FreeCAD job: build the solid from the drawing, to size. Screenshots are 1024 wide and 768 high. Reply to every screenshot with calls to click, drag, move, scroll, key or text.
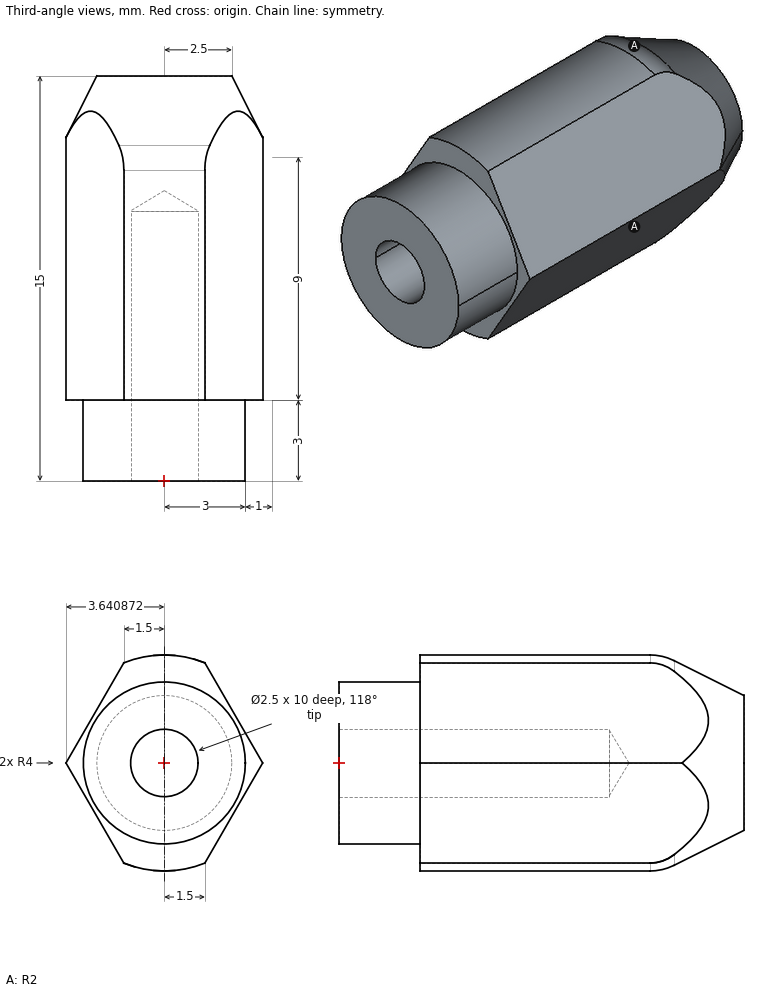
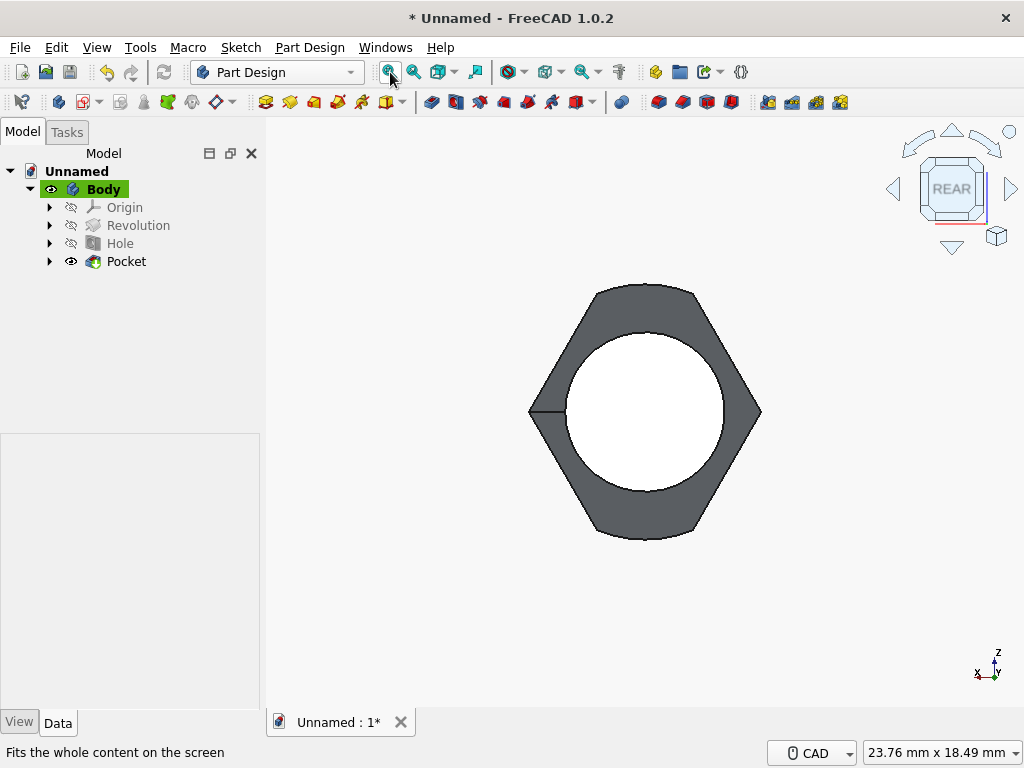
key(0)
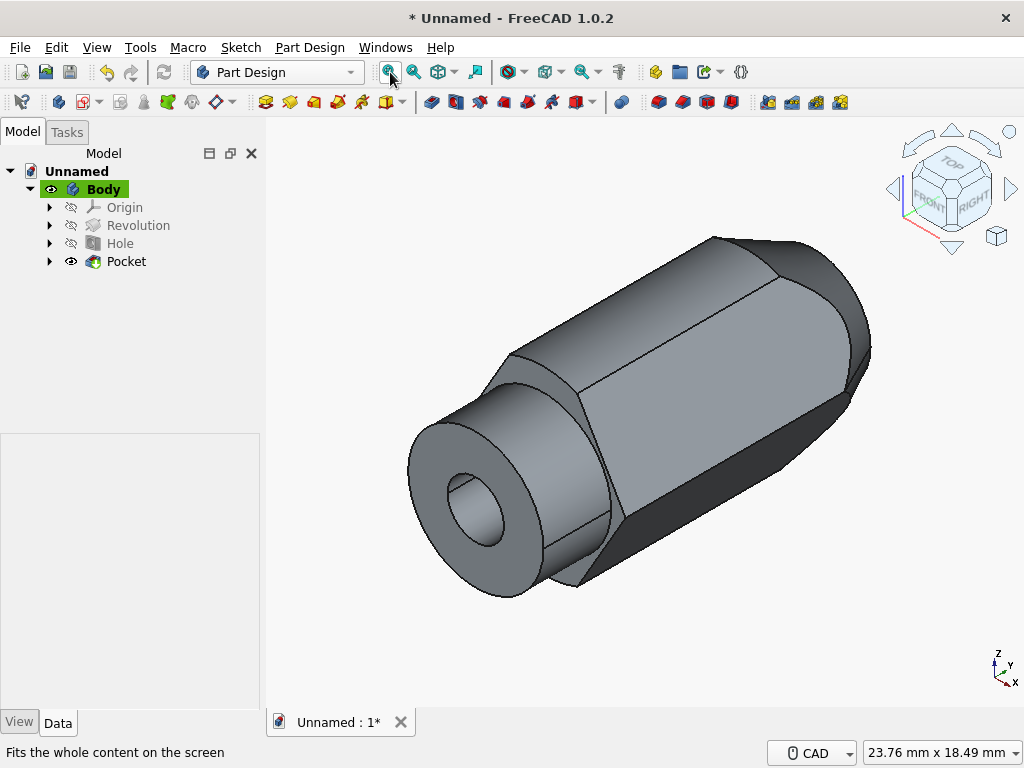
click(733, 241)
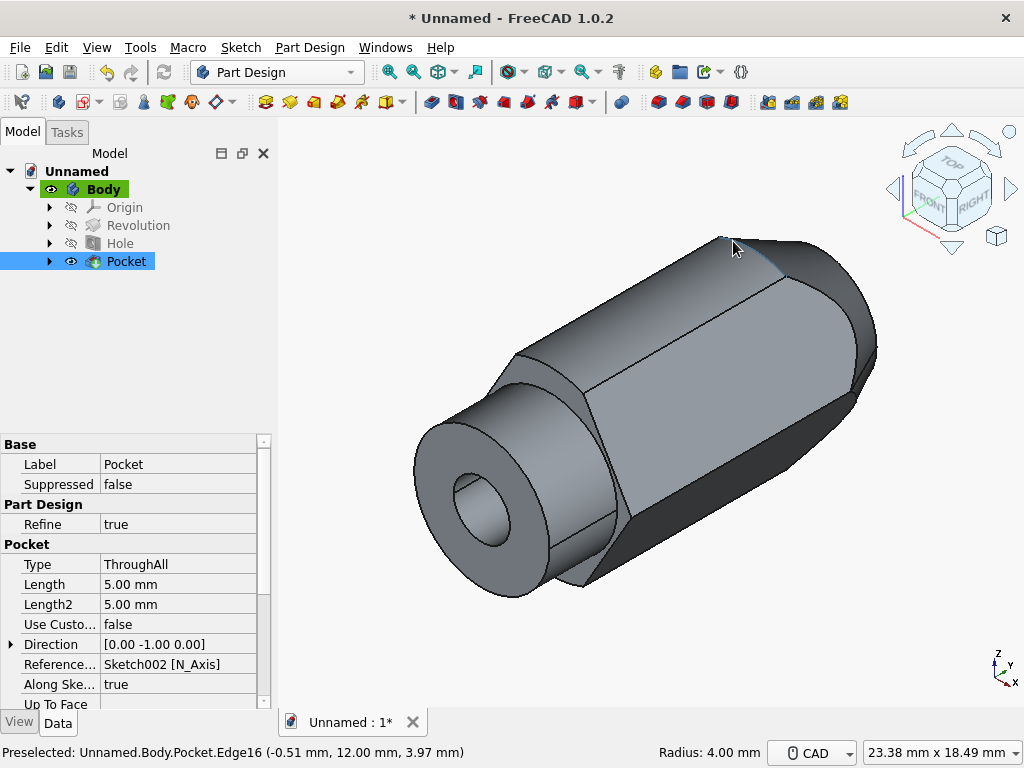
key(2)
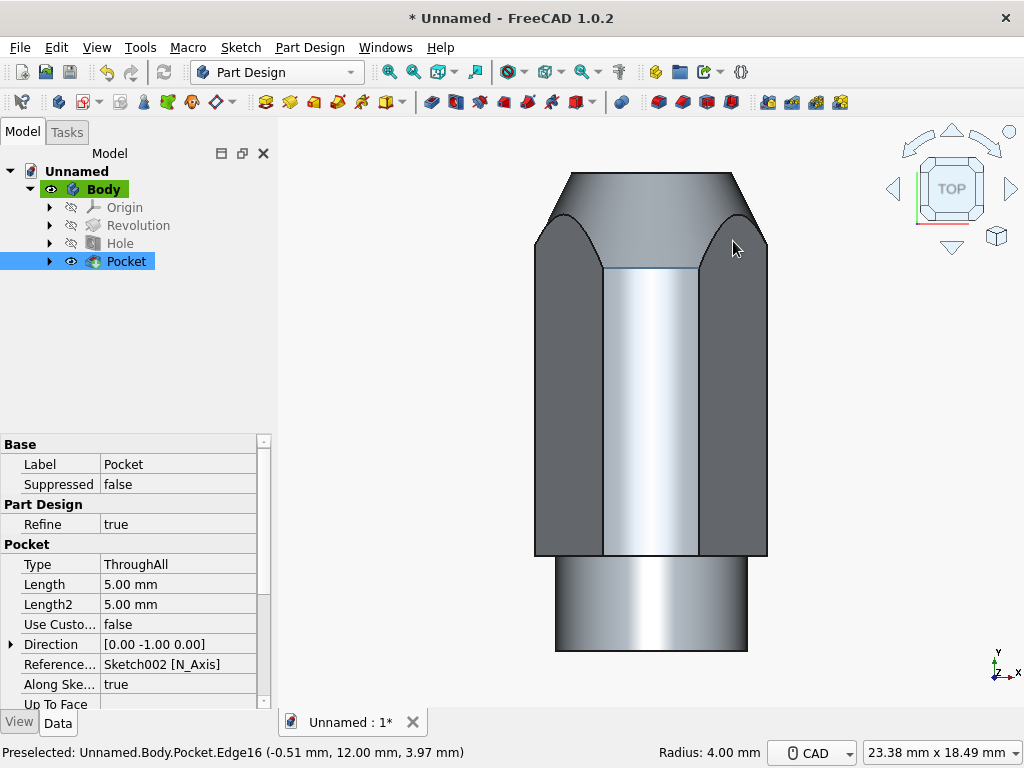
key(1)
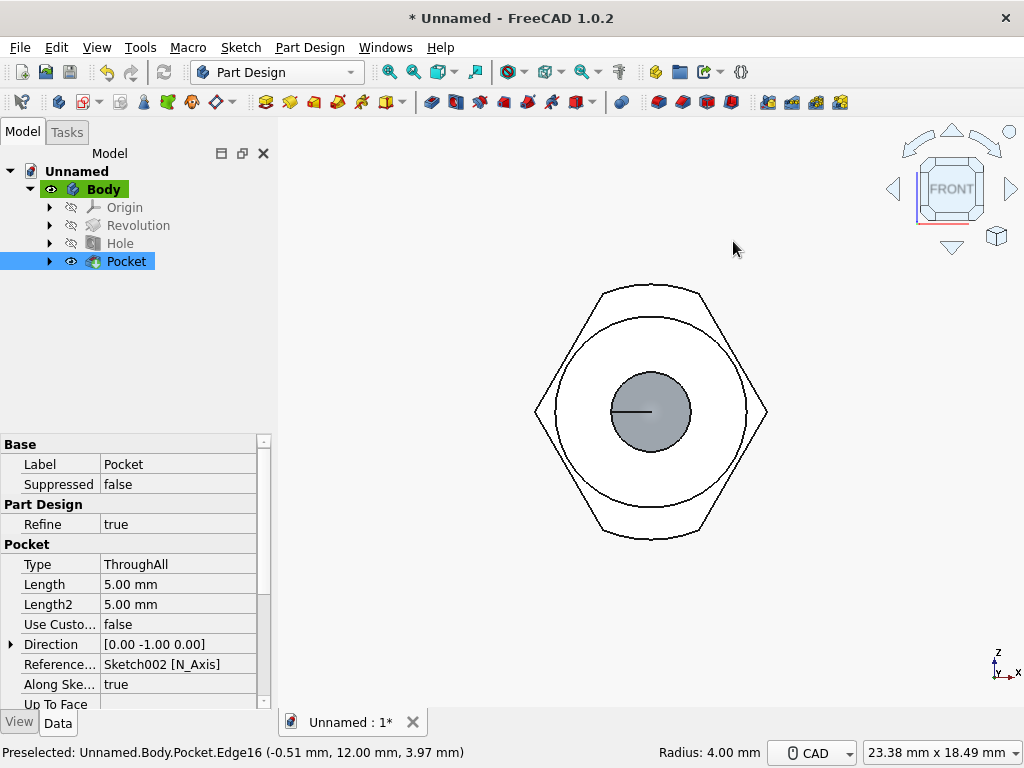
click(390, 72)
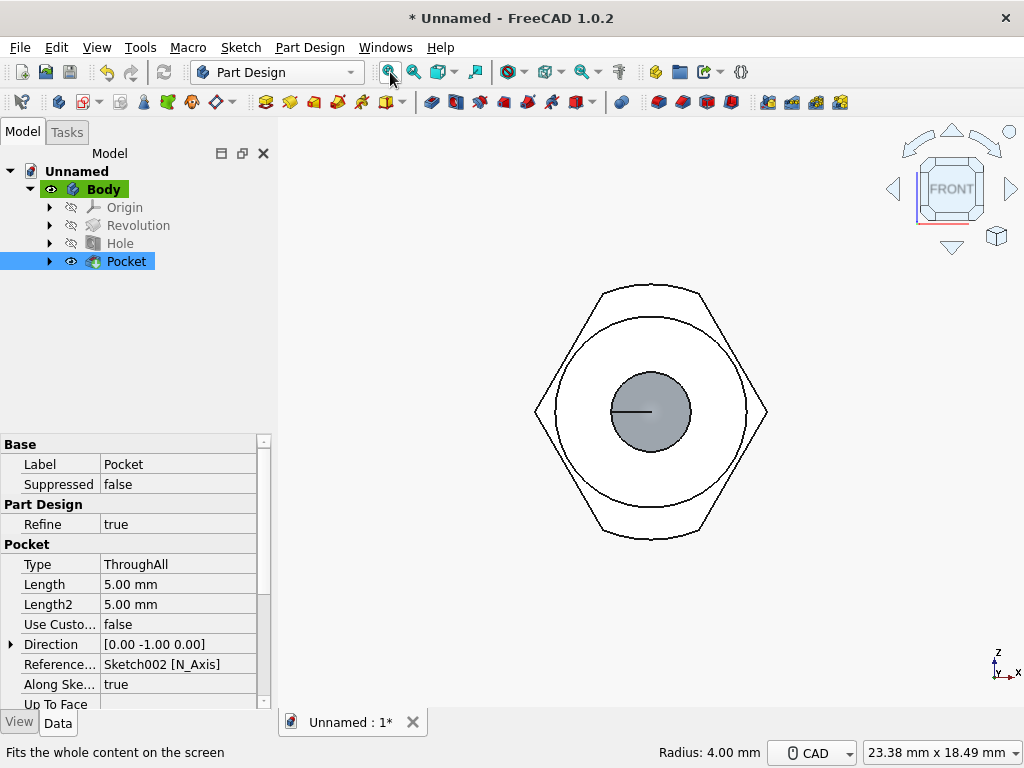
key(3)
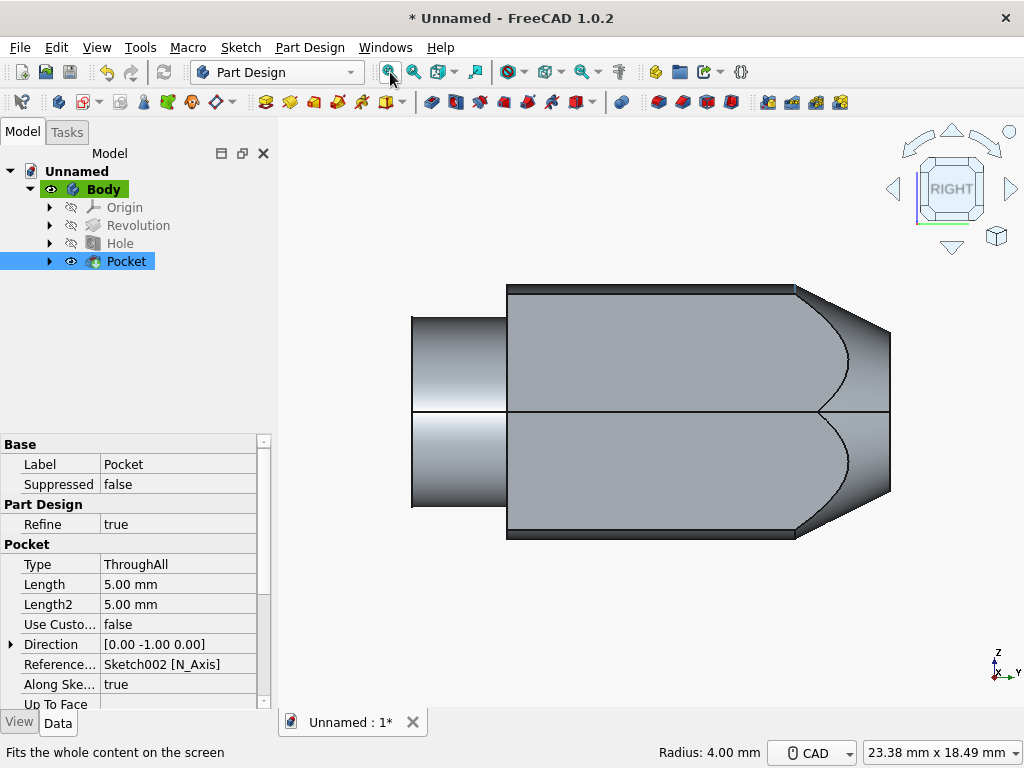
click(795, 537, ctrl)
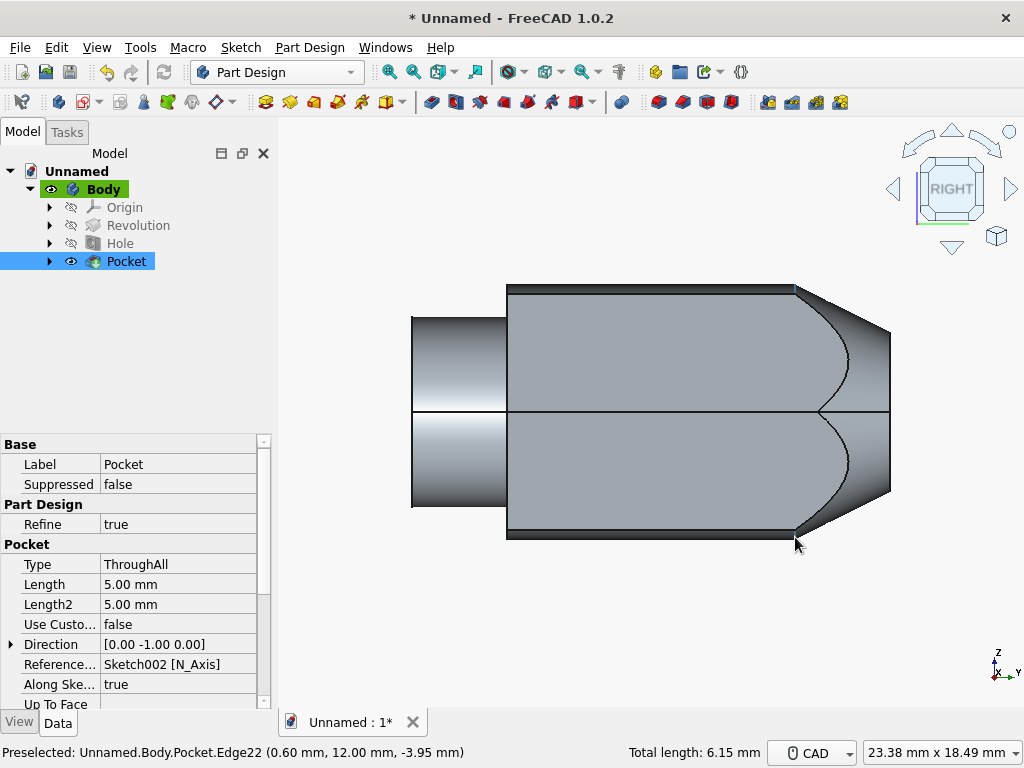
click(660, 102)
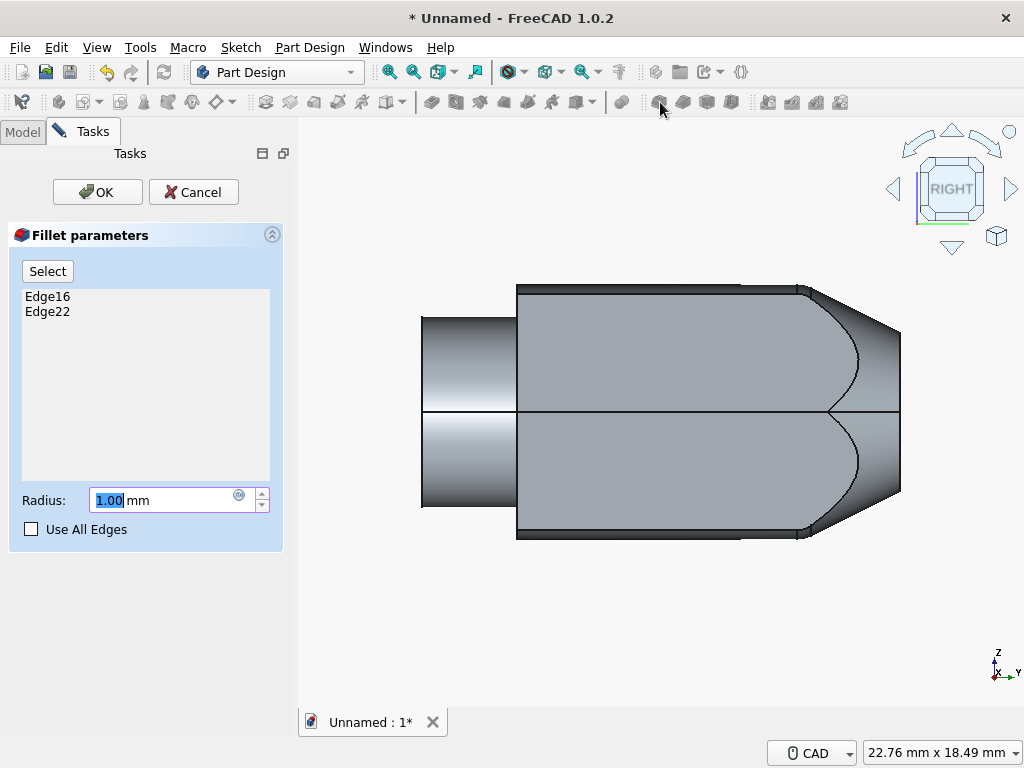
text(2)
key(Tab)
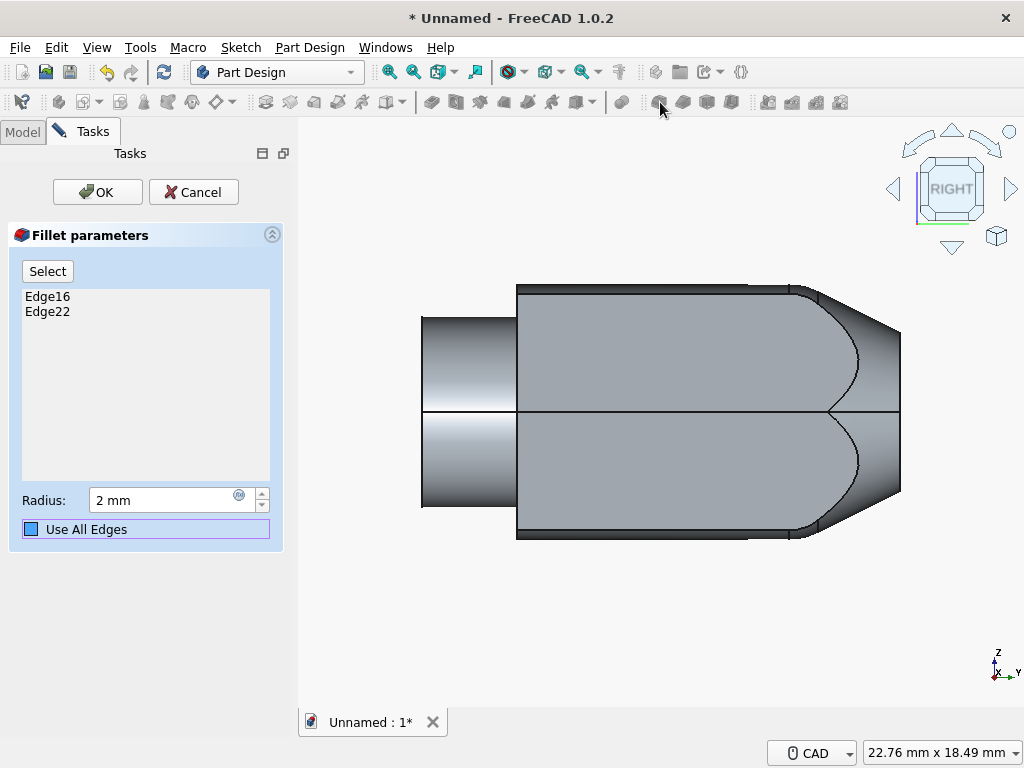
click(98, 192)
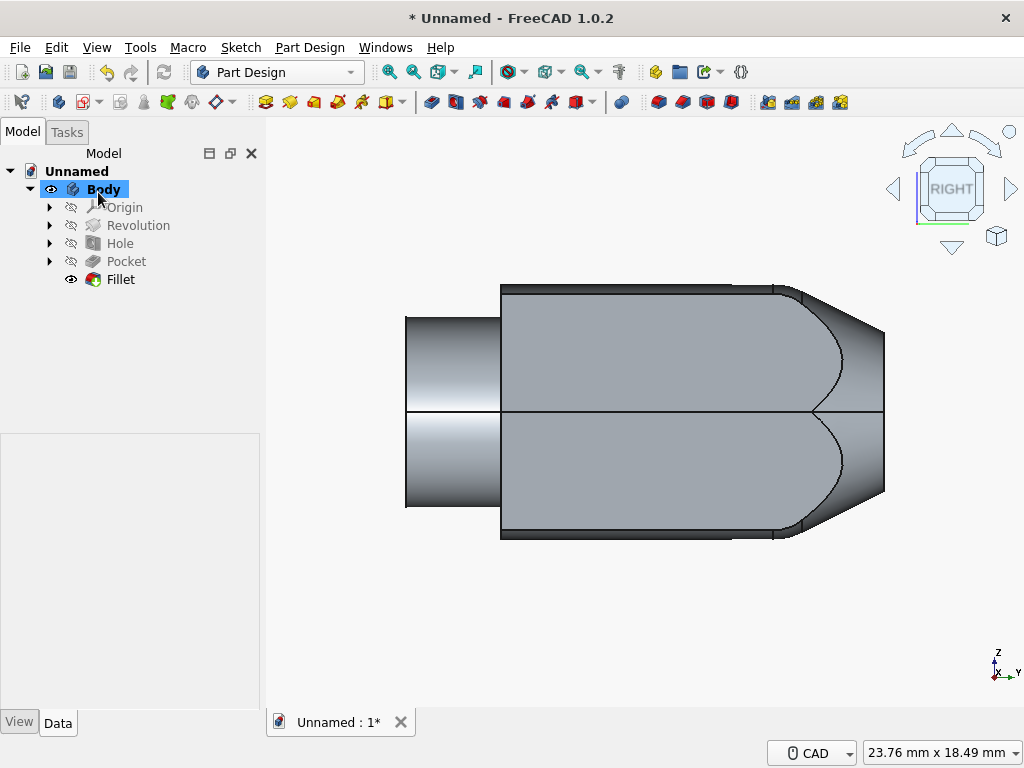
key(0)